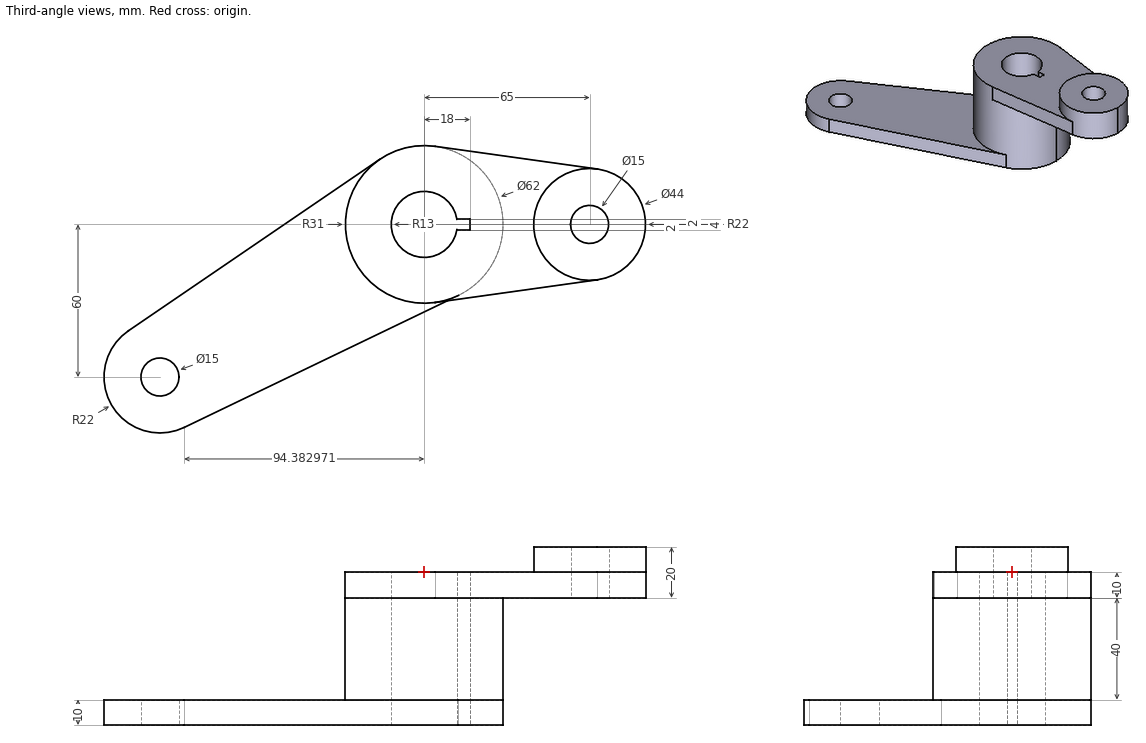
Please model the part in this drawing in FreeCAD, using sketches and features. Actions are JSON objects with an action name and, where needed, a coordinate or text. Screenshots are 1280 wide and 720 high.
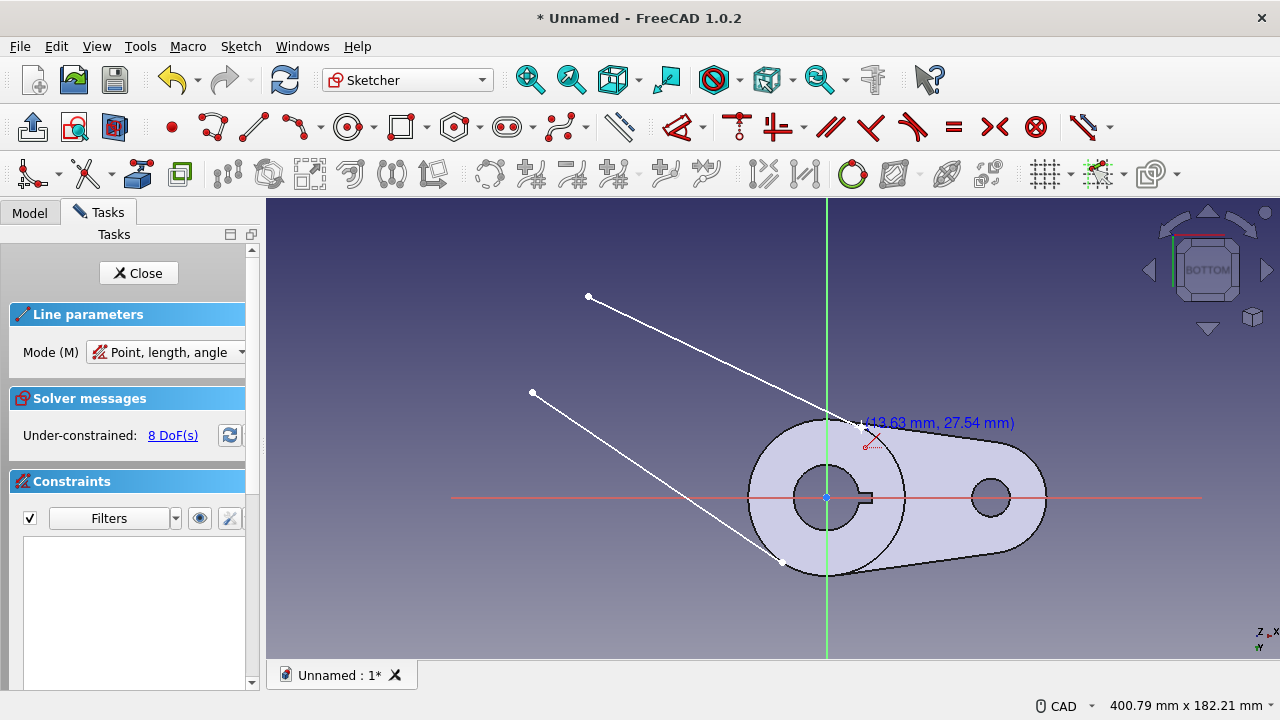
{"action": "key", "text": "g 3 a"}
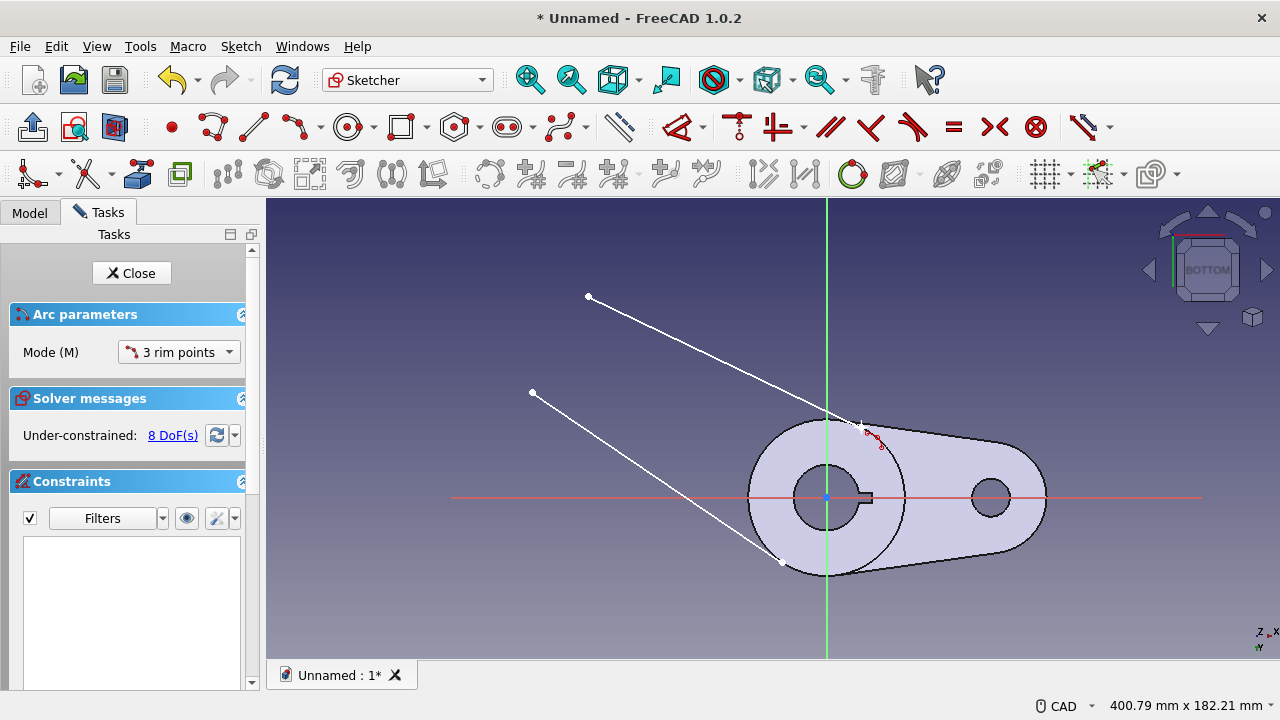
{"action": "left_click", "coordinate": [532, 393]}
{"action": "left_click", "coordinate": [588, 297]}
{"action": "left_click", "coordinate": [515, 318]}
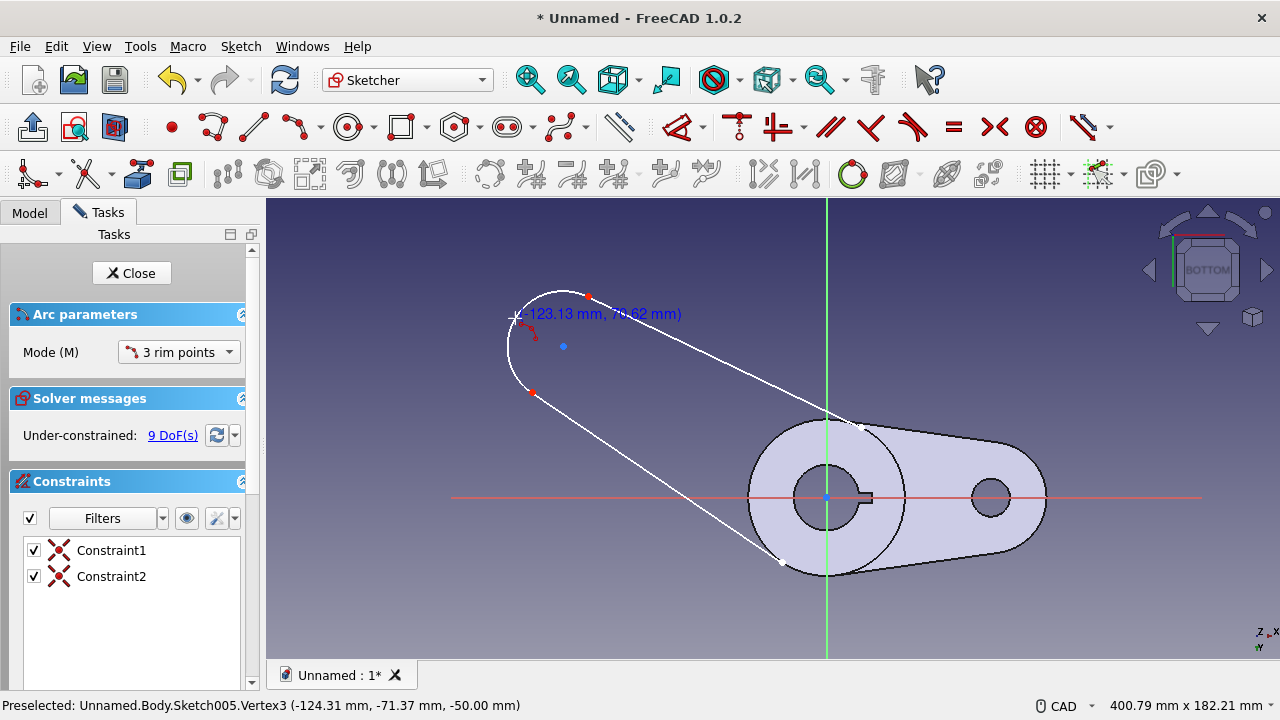
{"action": "left_click", "coordinate": [861, 428]}
{"action": "left_click", "coordinate": [782, 563]}
{"action": "left_click", "coordinate": [894, 537]}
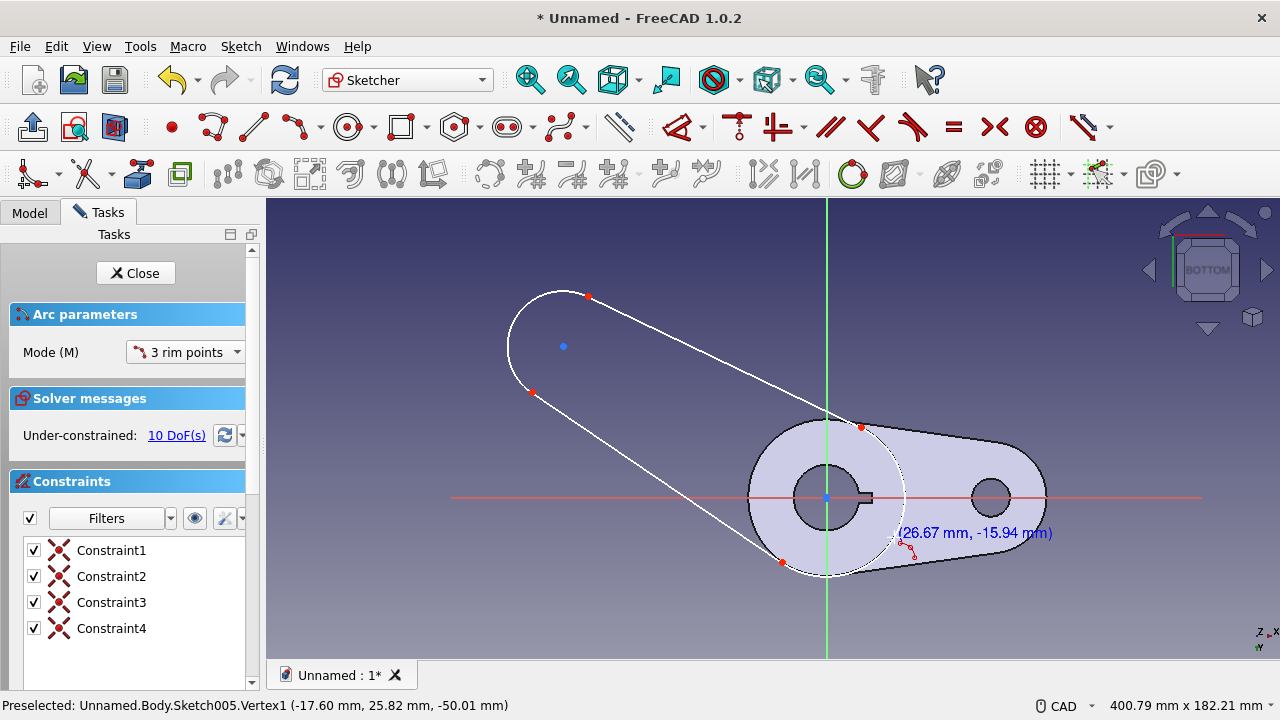
{"action": "left_click", "coordinate": [213, 128]}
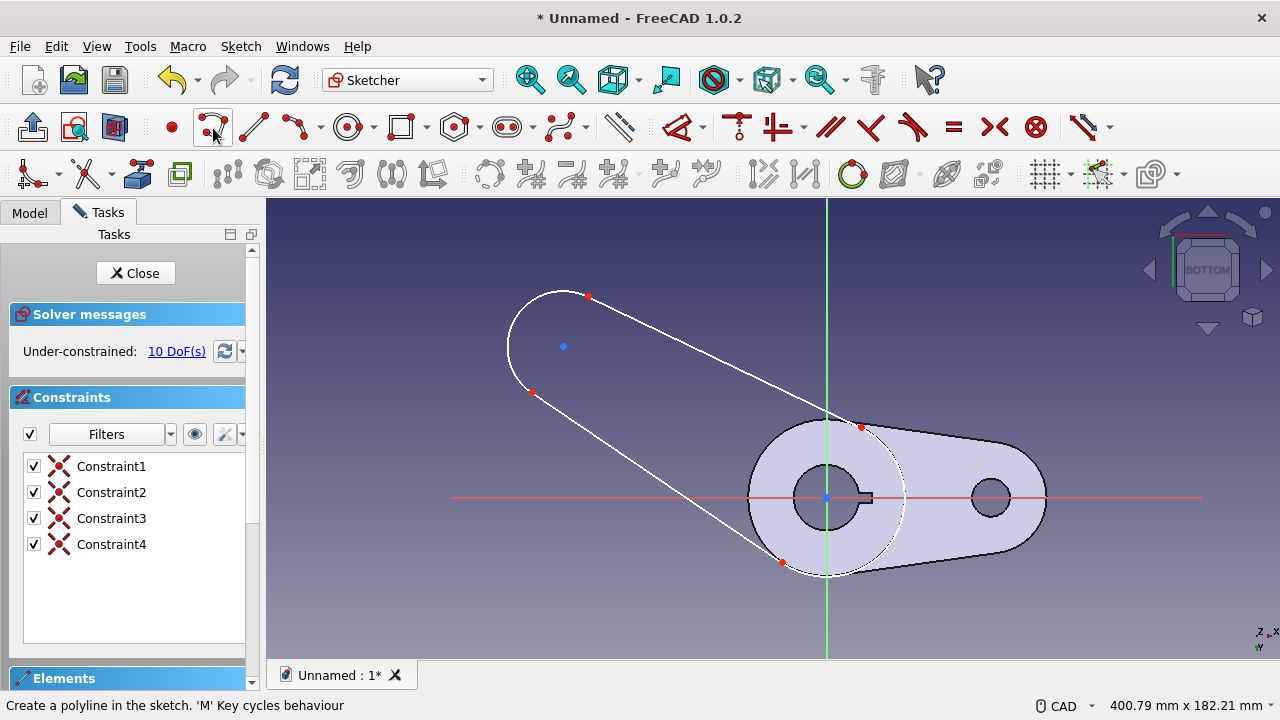
{"action": "scroll", "coordinate": [859, 503], "scroll_direction": "up", "scroll_amount": 6}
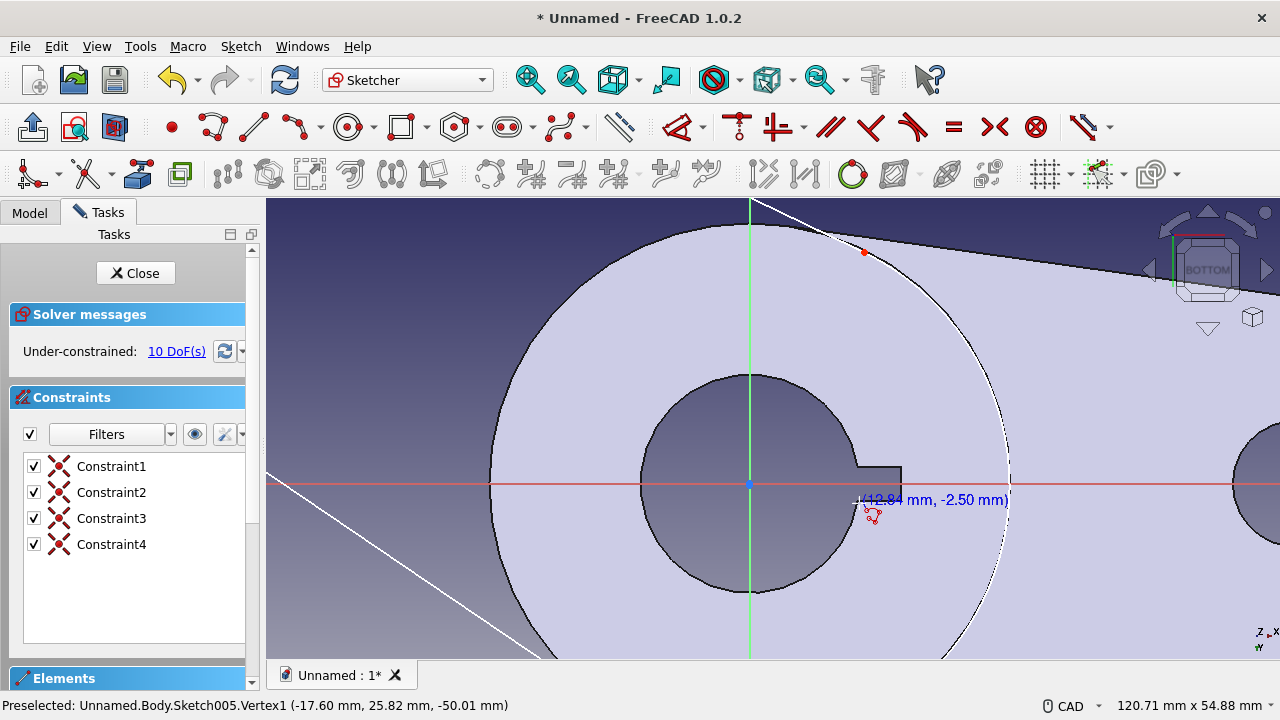
{"action": "left_click", "coordinate": [858, 501]}
{"action": "left_click", "coordinate": [901, 501]}
{"action": "left_click", "coordinate": [901, 467]}
{"action": "left_click", "coordinate": [858, 467]}
{"action": "right_click", "coordinate": [858, 467]}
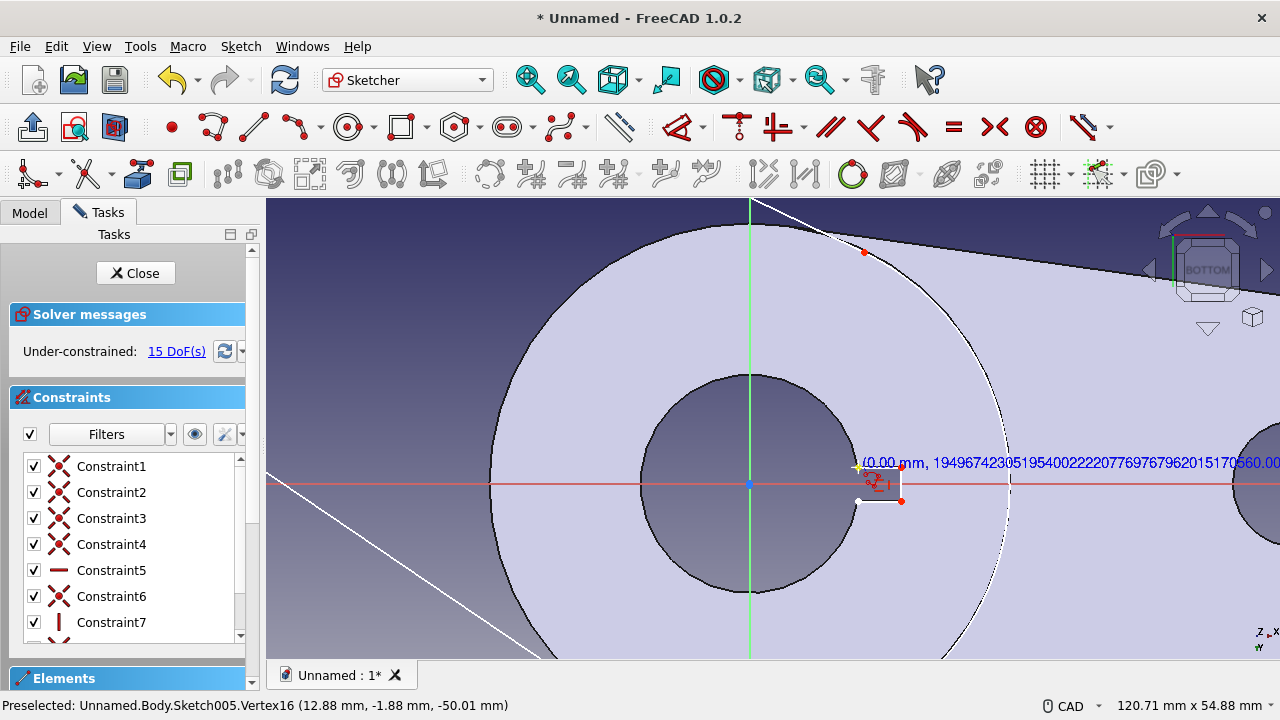
{"action": "left_click", "coordinate": [294, 128]}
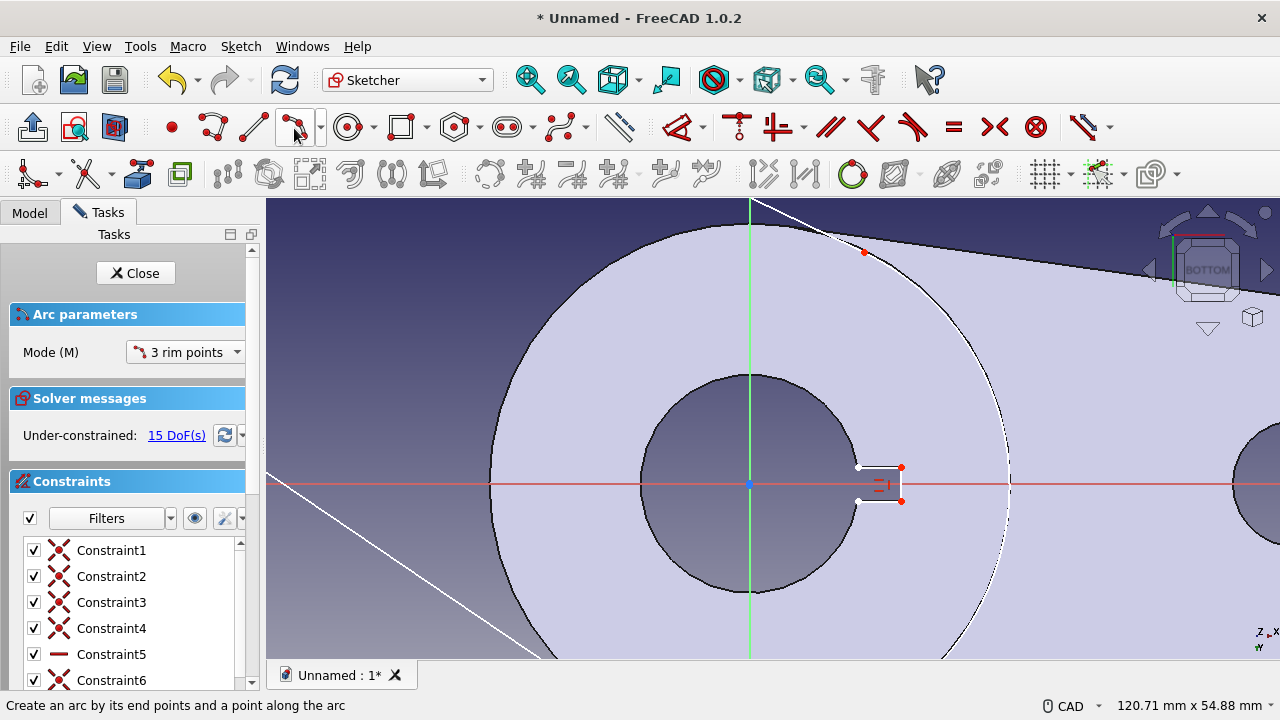
{"action": "left_click", "coordinate": [858, 468]}
{"action": "left_click", "coordinate": [858, 502]}
{"action": "left_click", "coordinate": [660, 422]}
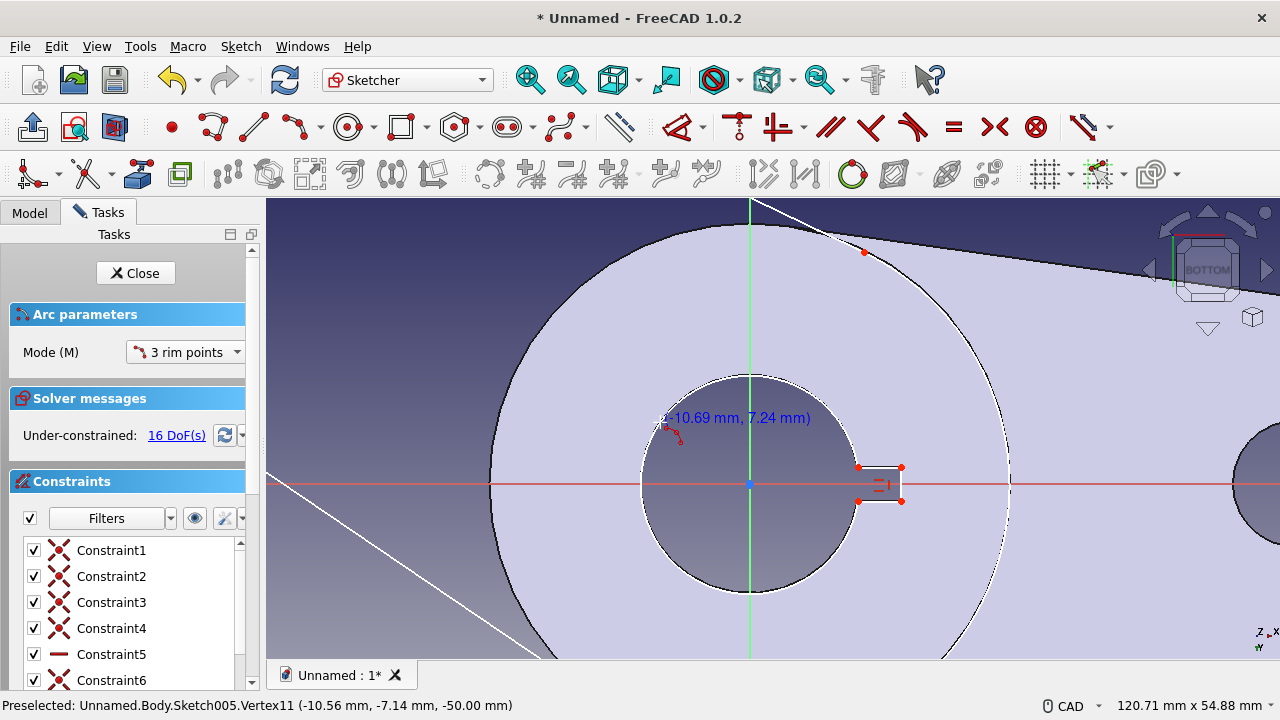
{"action": "key", "text": "g c"}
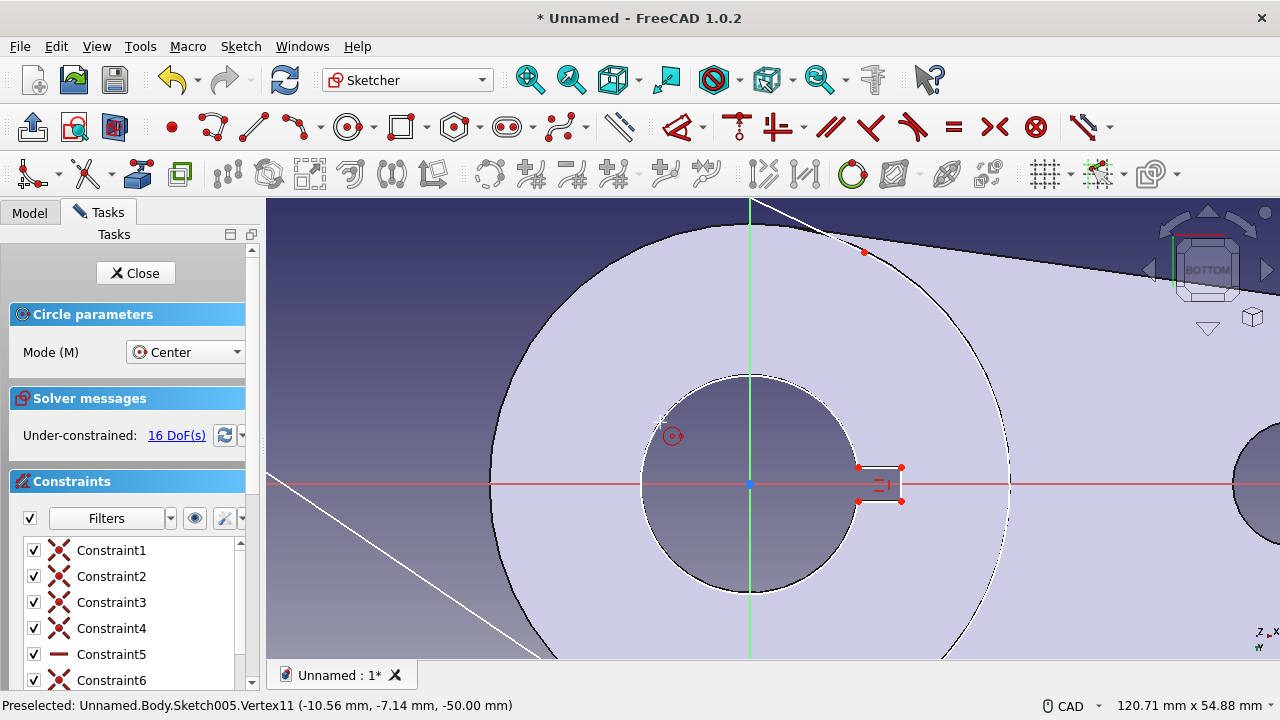
{"action": "scroll", "coordinate": [859, 503], "scroll_direction": "down", "scroll_amount": 6}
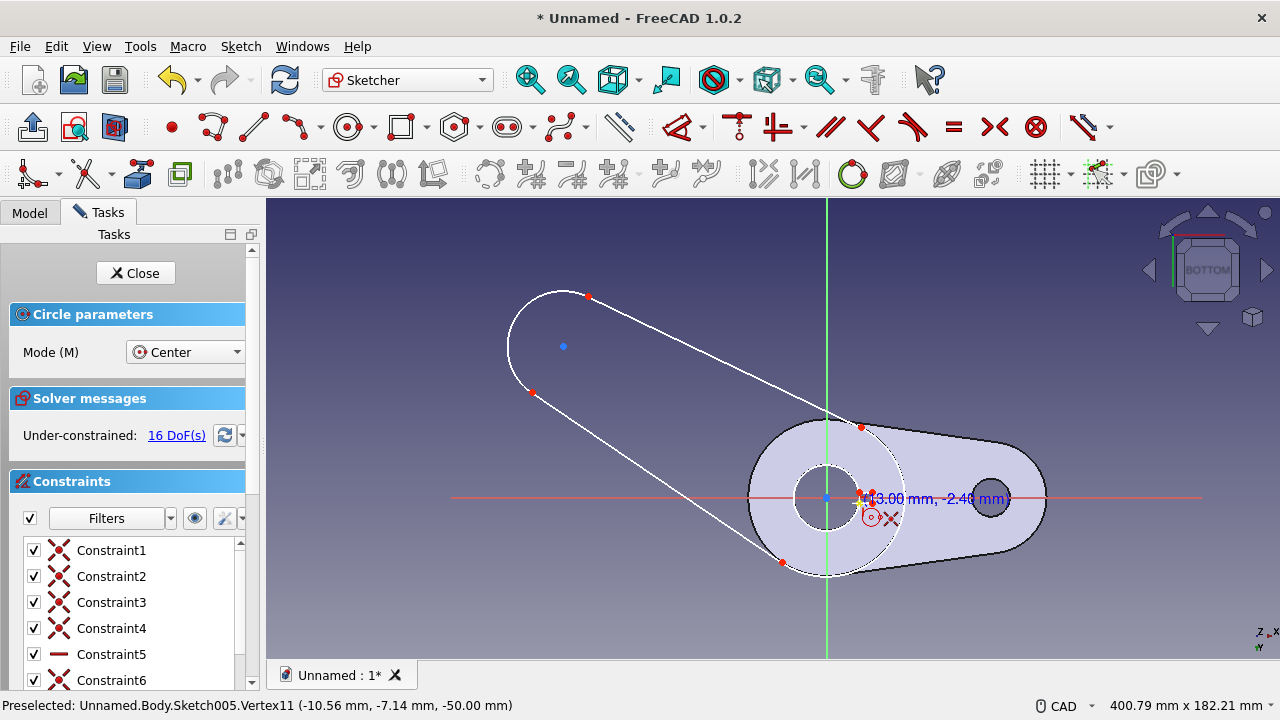
{"action": "left_click", "coordinate": [564, 346]}
{"action": "left_click", "coordinate": [577, 332]}
{"action": "key", "text": "Escape"}